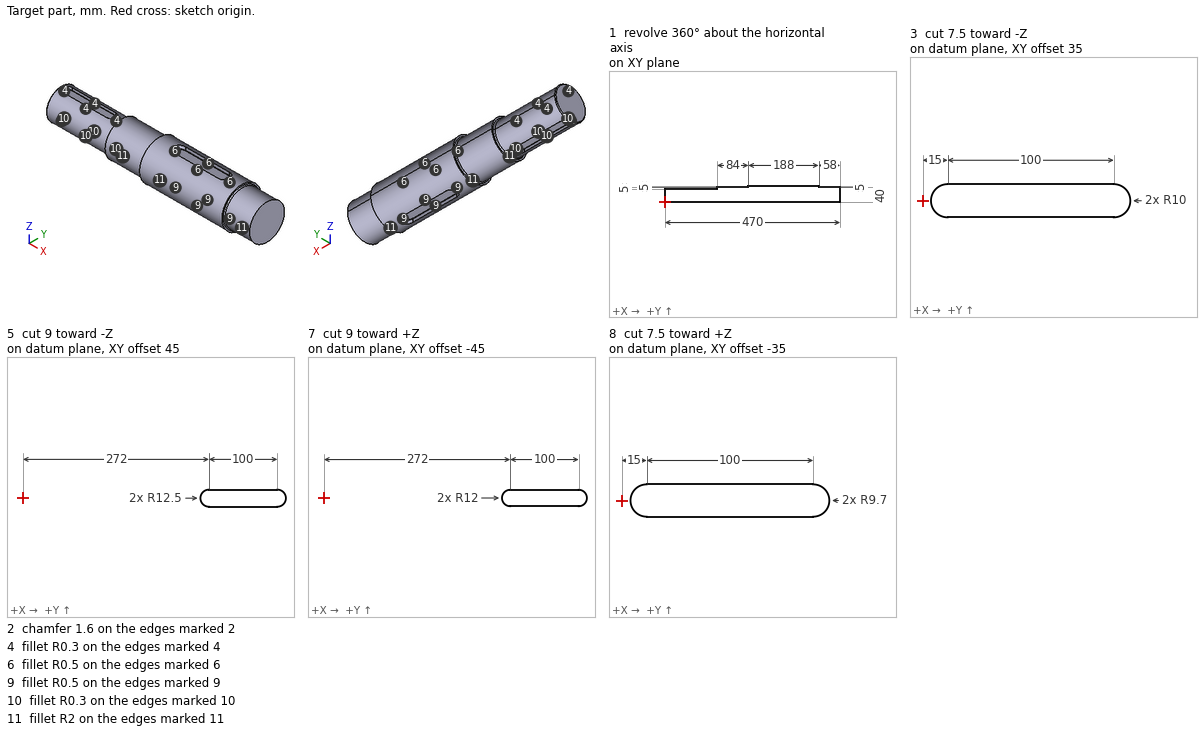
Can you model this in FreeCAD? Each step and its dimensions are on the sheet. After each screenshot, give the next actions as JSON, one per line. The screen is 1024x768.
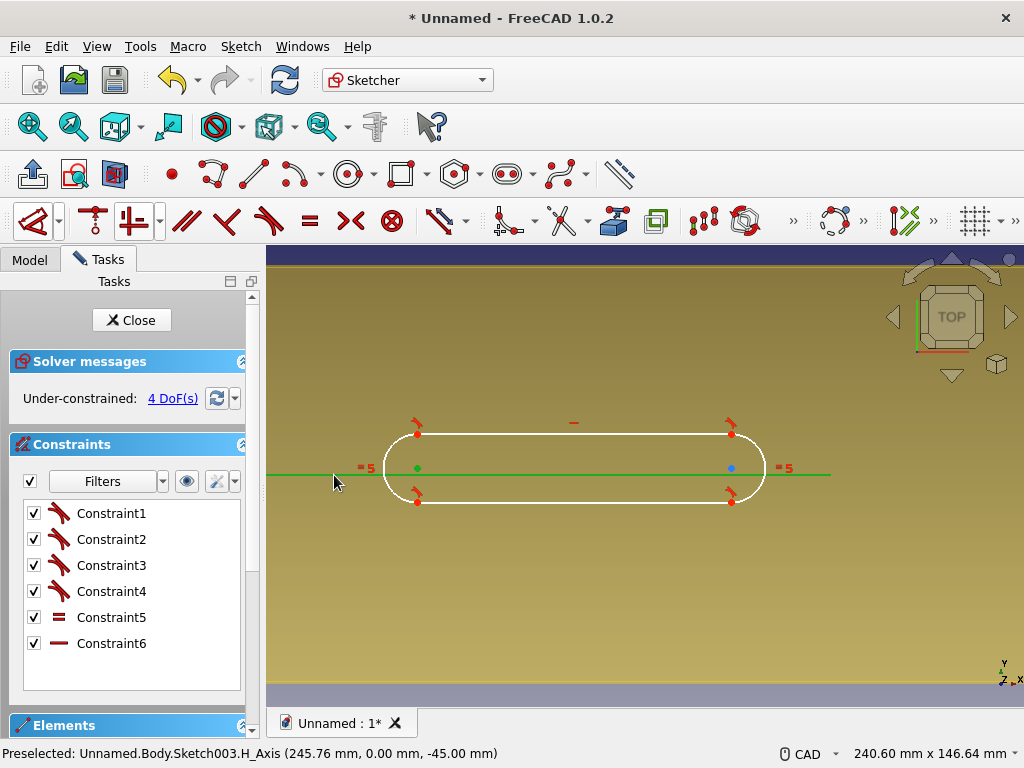
{"action": "left_click", "coordinate": [93, 222]}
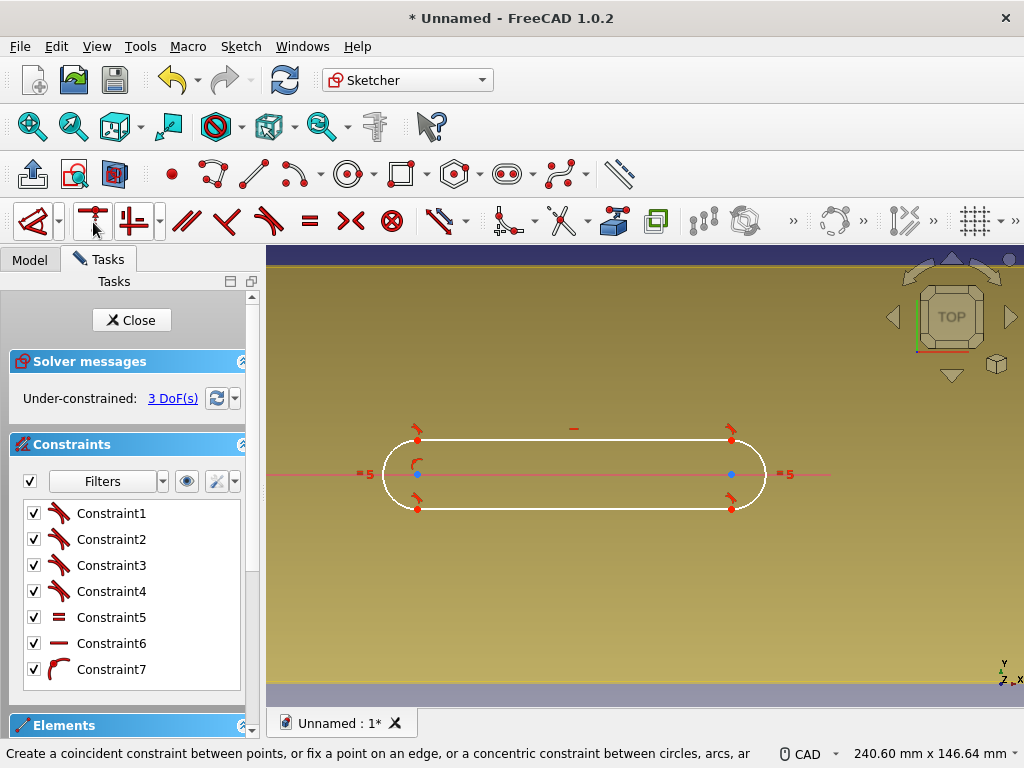
{"action": "left_click", "coordinate": [390, 455]}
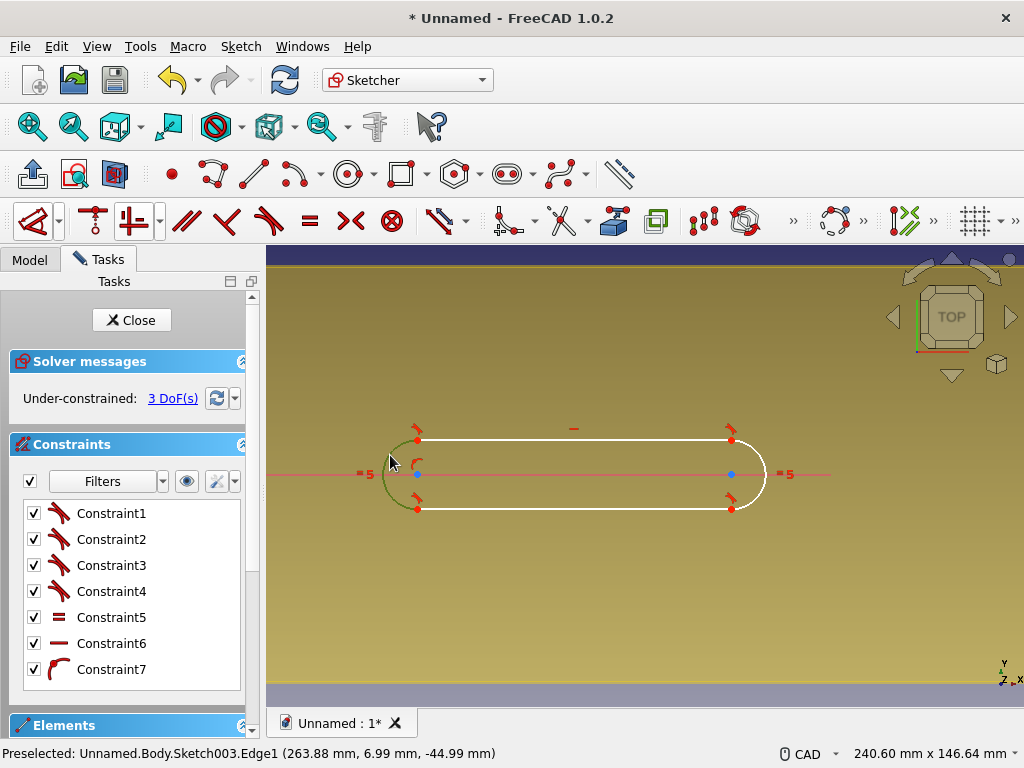
{"action": "key", "text": "k r"}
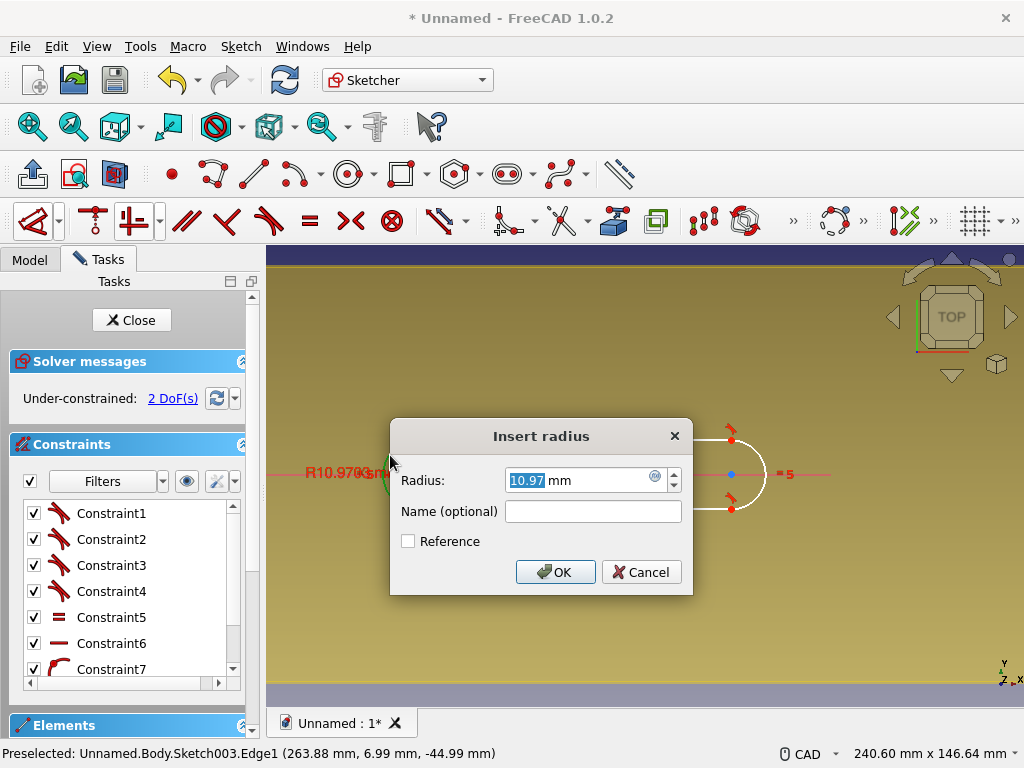
{"action": "type", "text": "12"}
{"action": "key", "text": "Return"}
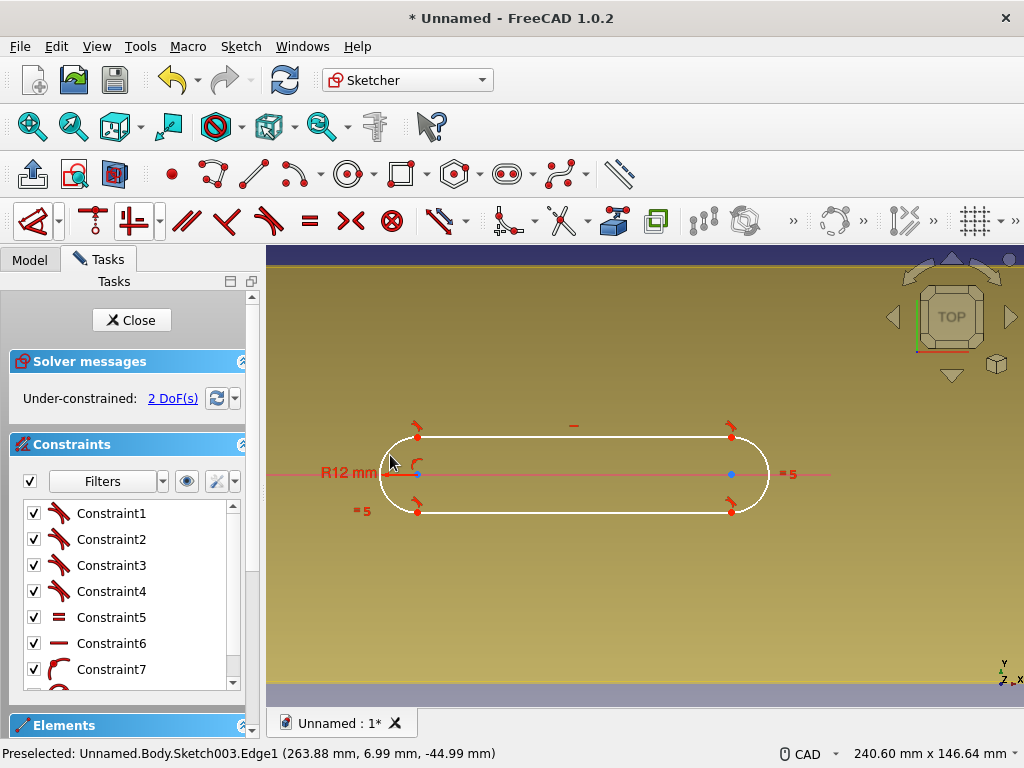
{"action": "left_click", "coordinate": [512, 437]}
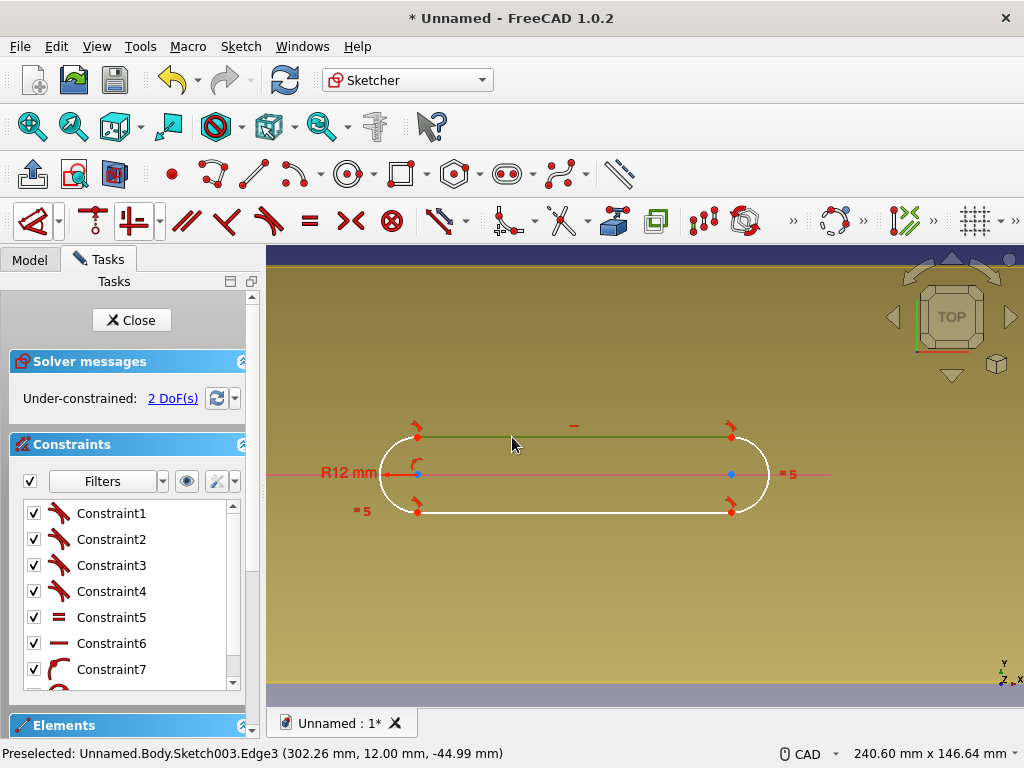
{"action": "left_click", "coordinate": [58, 222]}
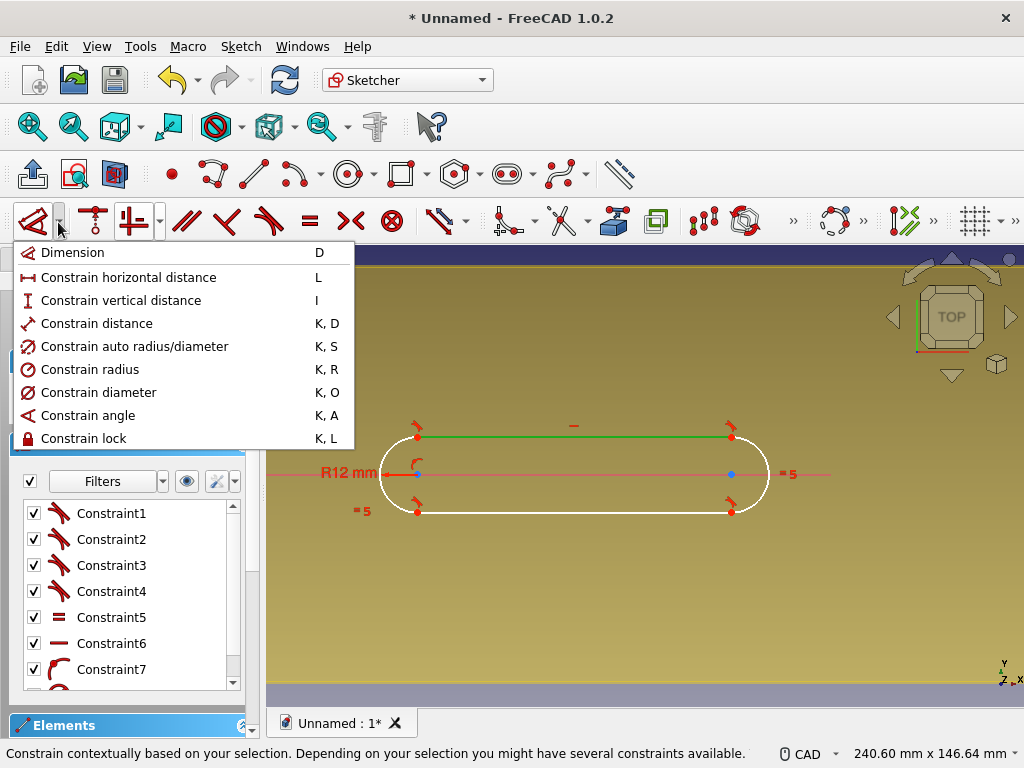
{"action": "left_click", "coordinate": [184, 278]}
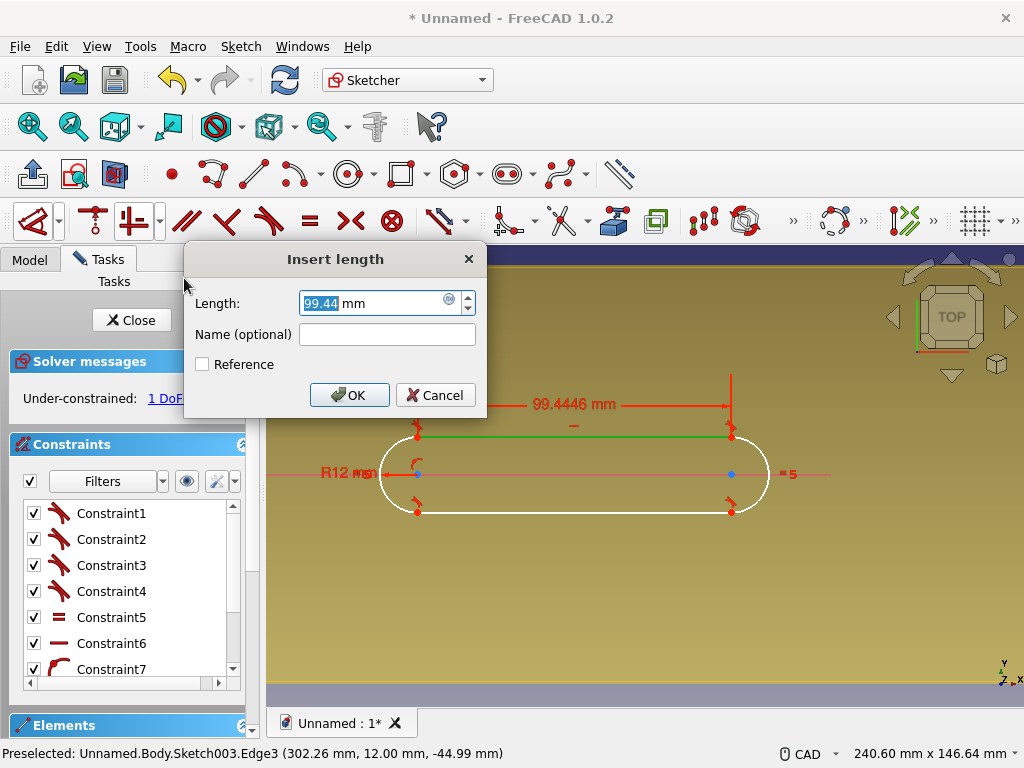
{"action": "type", "text": "100"}
{"action": "key", "text": "Return"}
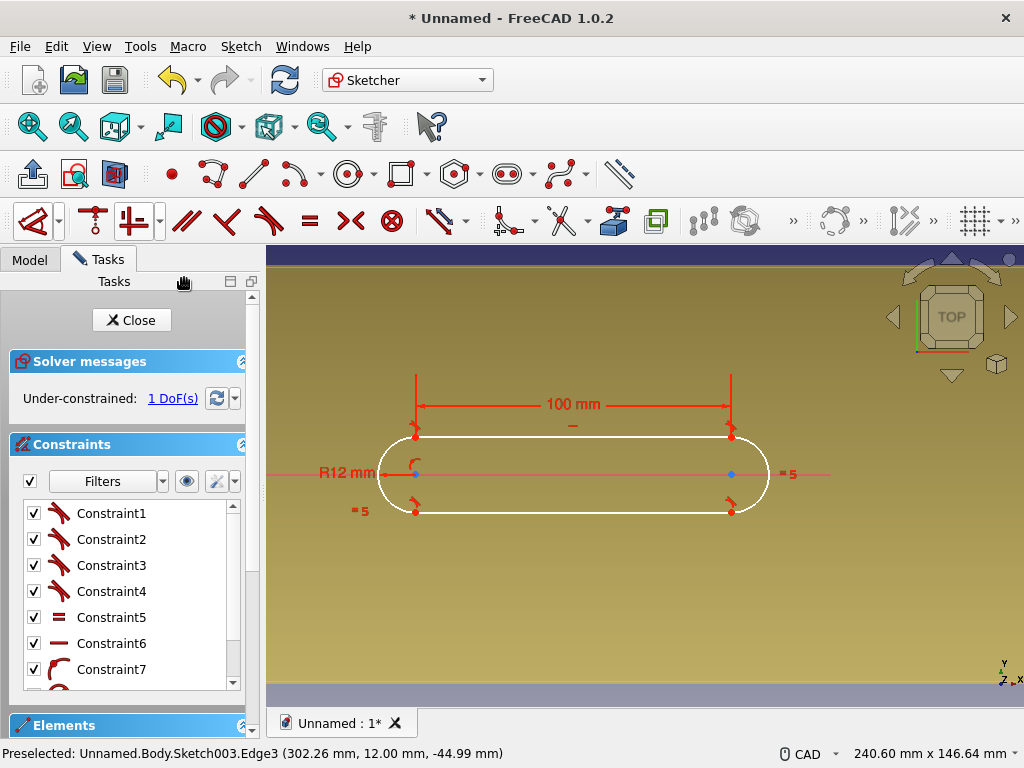
{"action": "left_click", "coordinate": [416, 437]}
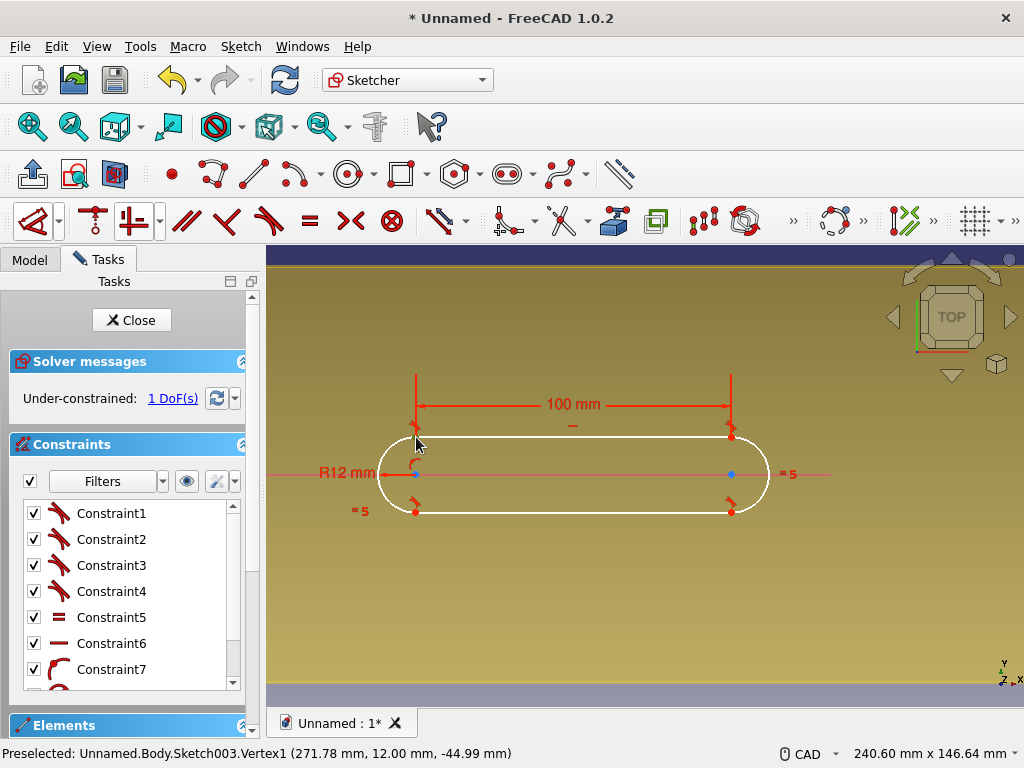
{"action": "key", "text": "l"}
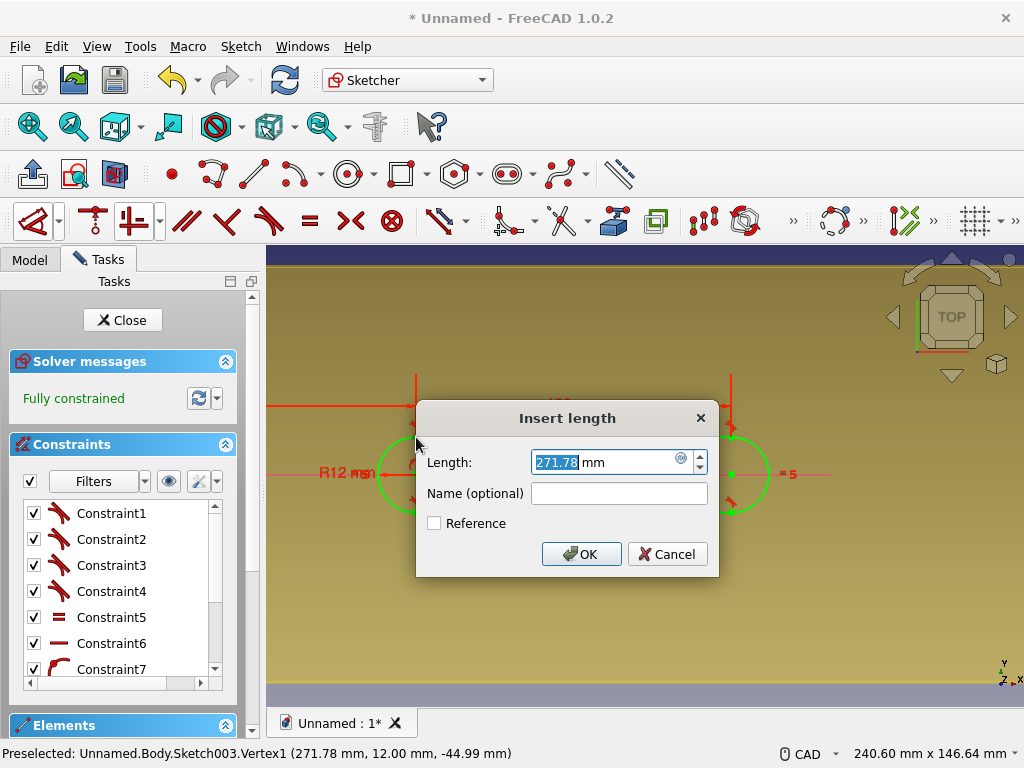
{"action": "type", "text": "272"}
{"action": "key", "text": "Return"}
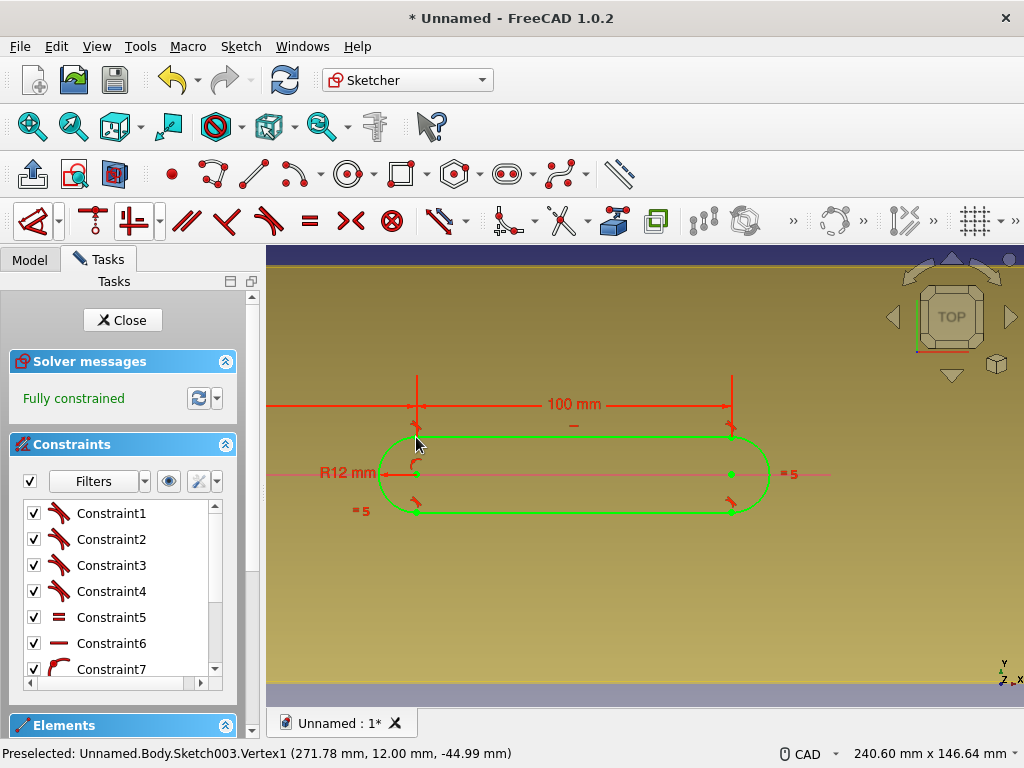
{"action": "left_click", "coordinate": [123, 320]}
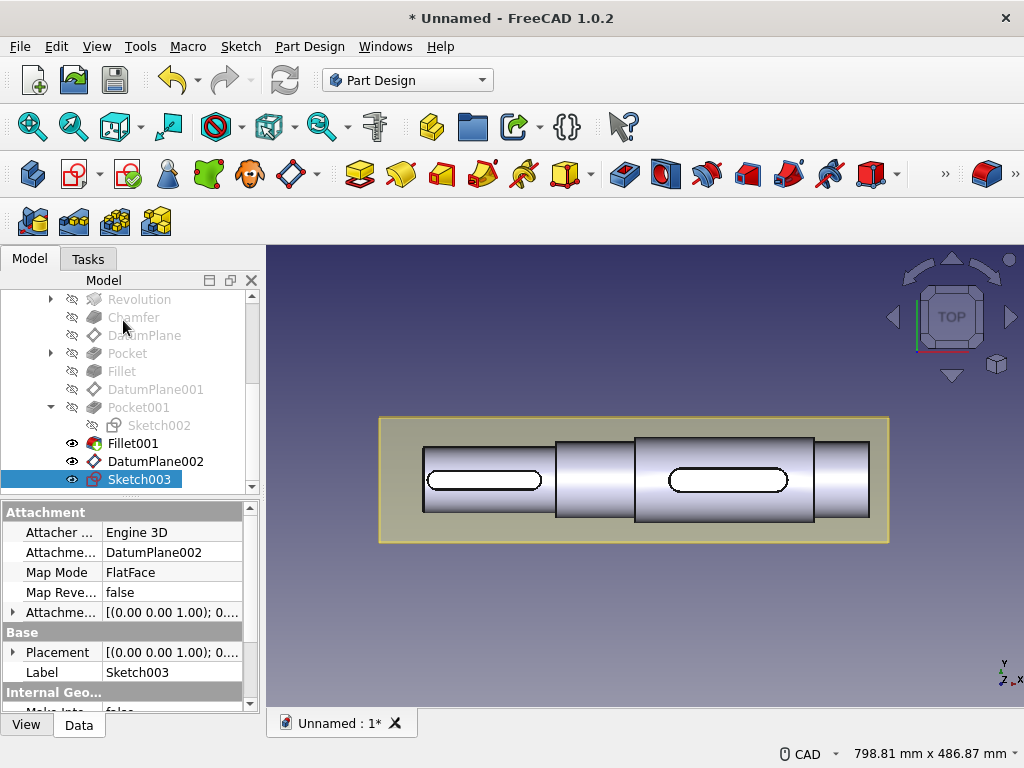
{"action": "left_click", "coordinate": [625, 174]}